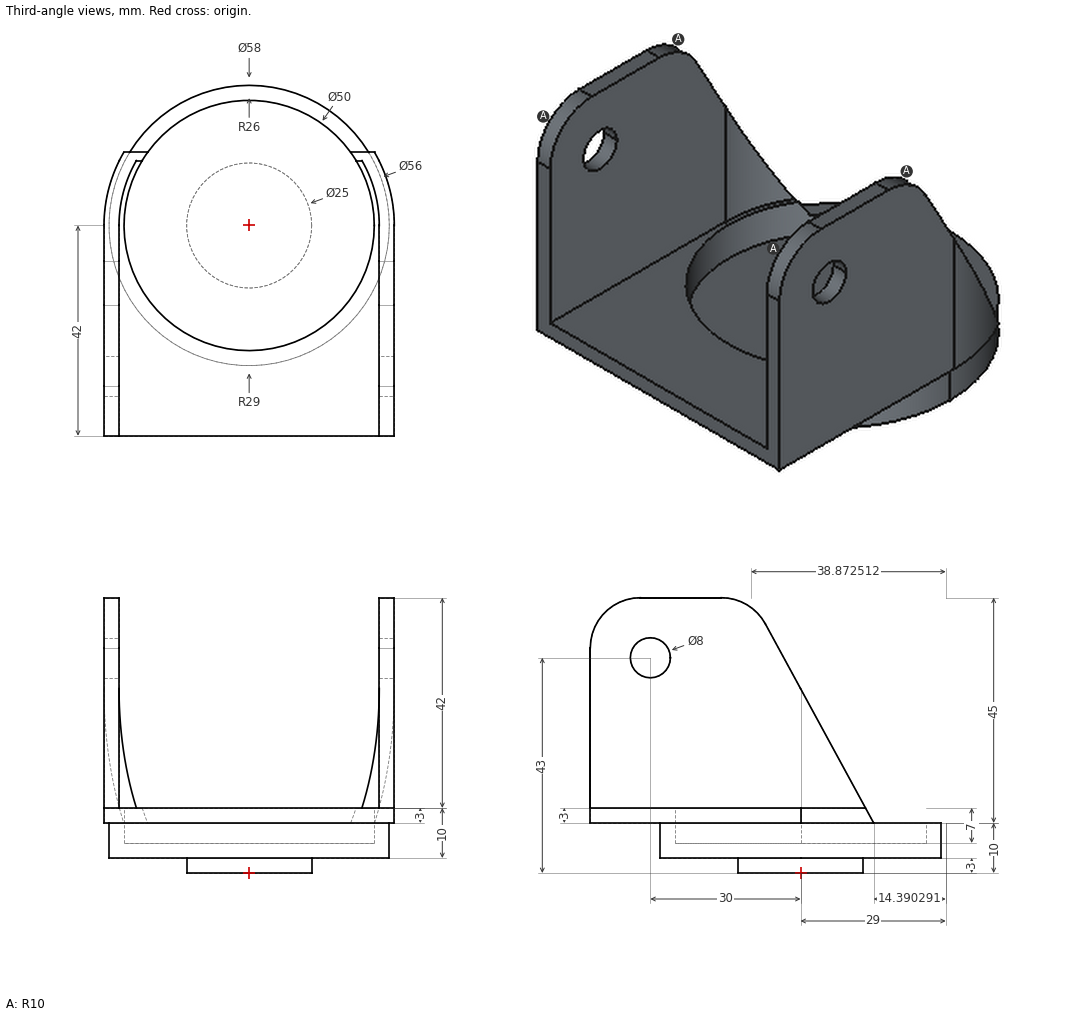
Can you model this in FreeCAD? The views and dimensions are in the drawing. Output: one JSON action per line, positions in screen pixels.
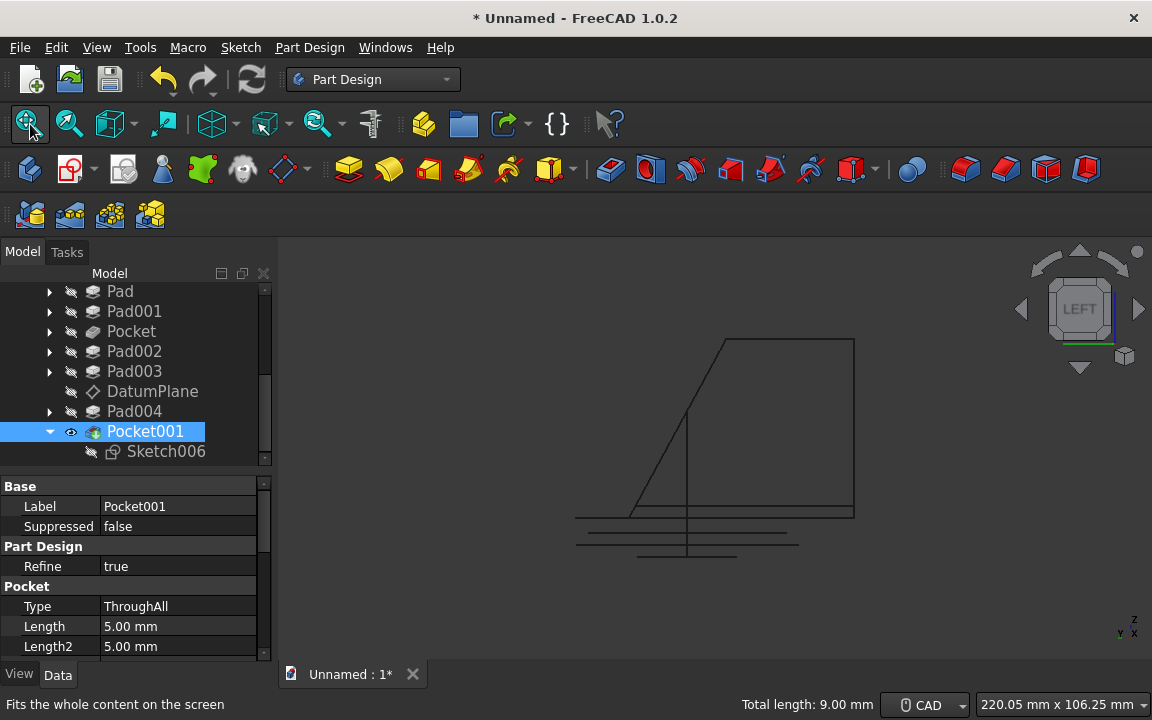
{"action": "key", "text": "0"}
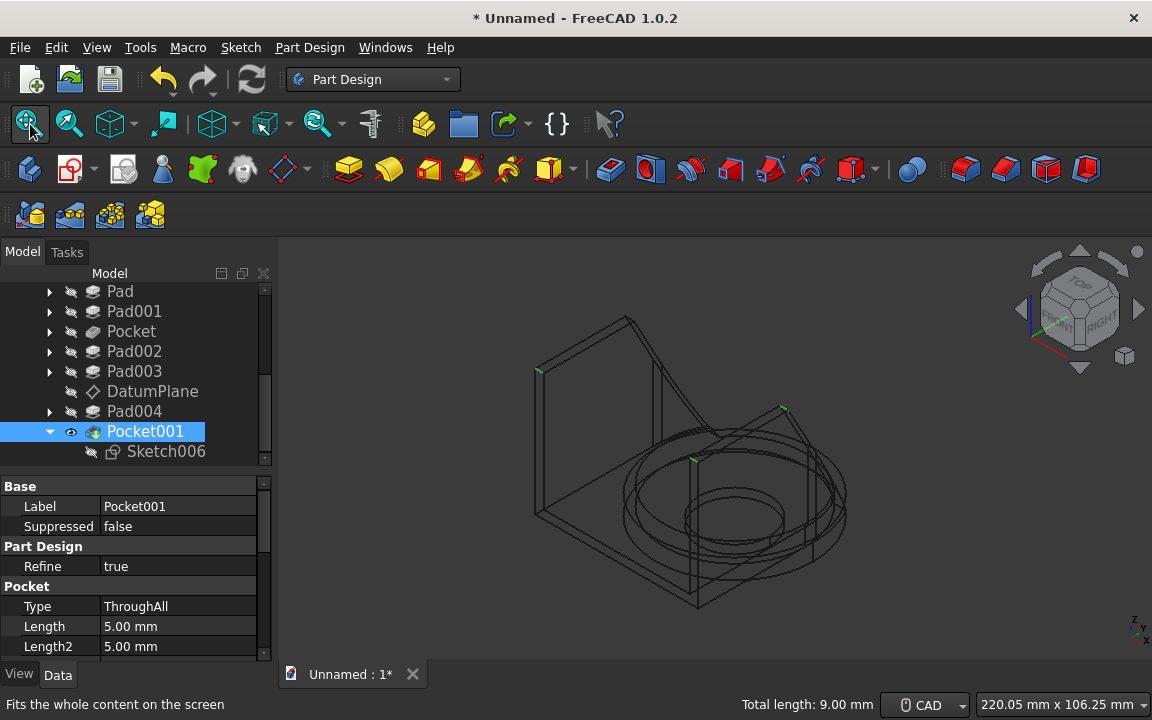
{"action": "left_click", "coordinate": [627, 316], "text": "ctrl"}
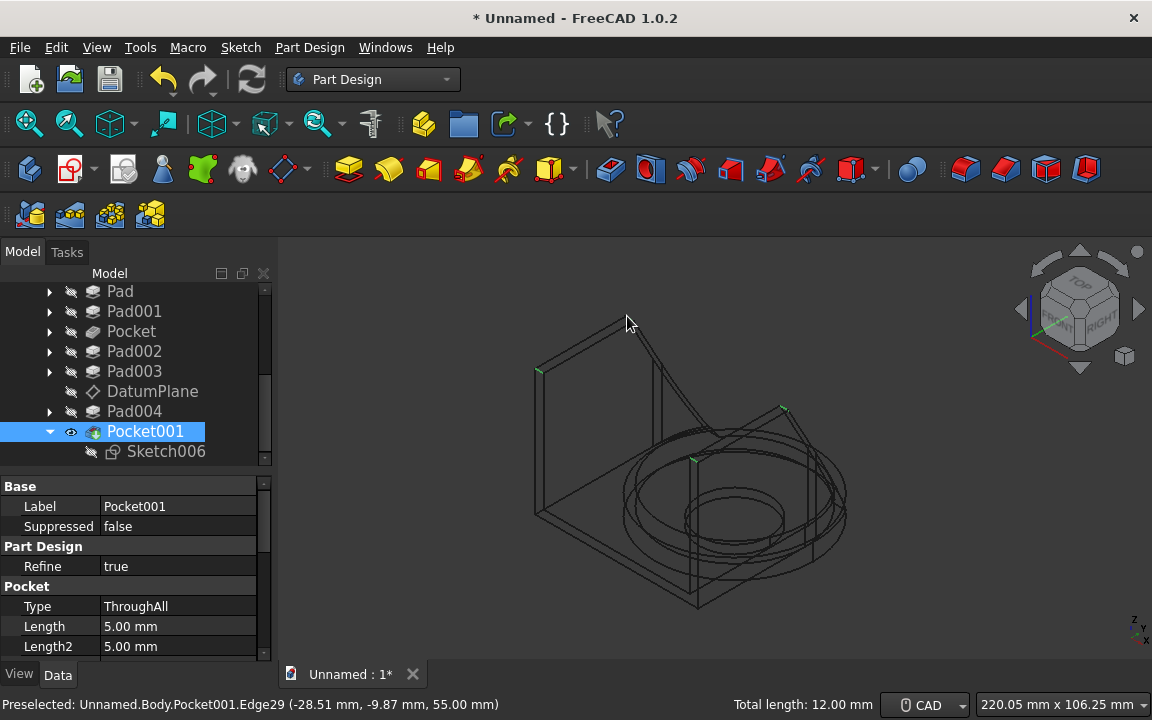
{"action": "key", "text": "v 1"}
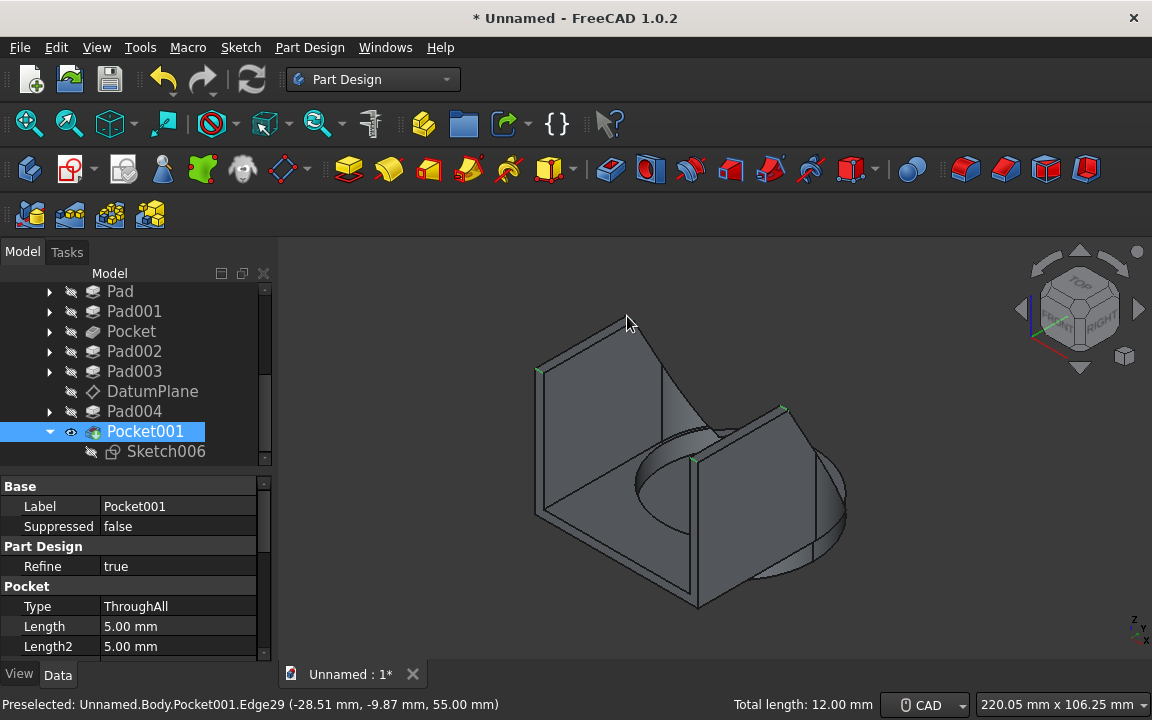
{"action": "left_click", "coordinate": [966, 170]}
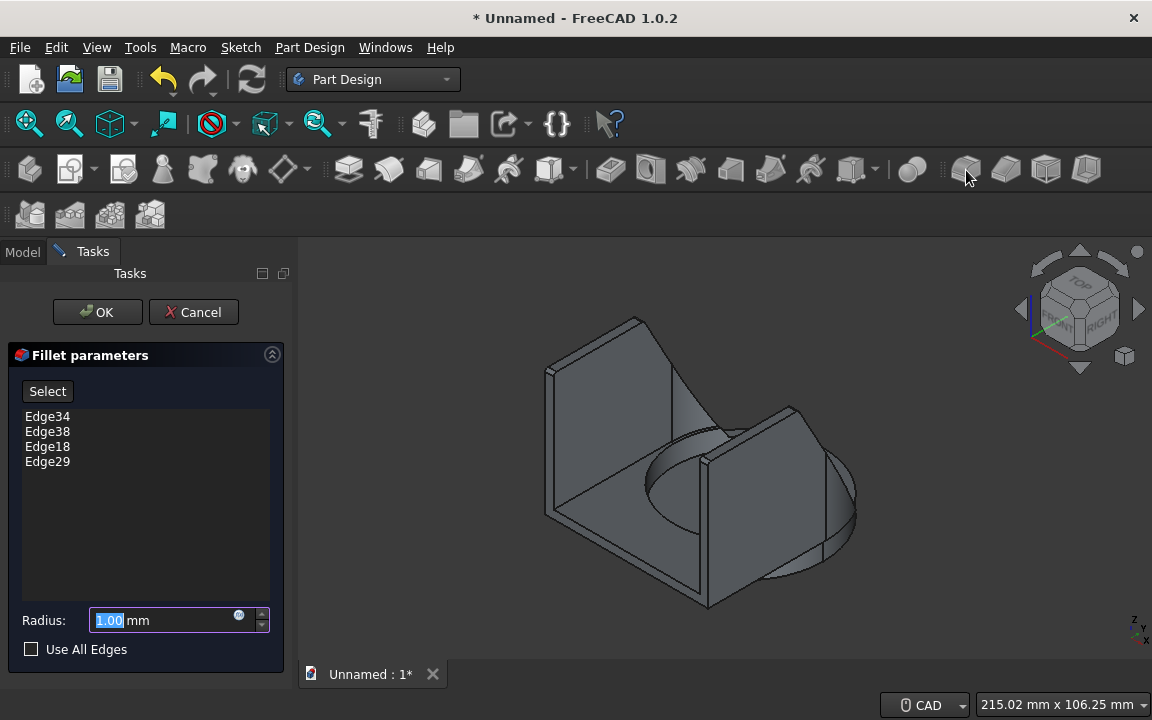
{"action": "type", "text": "10"}
{"action": "key", "text": "Tab"}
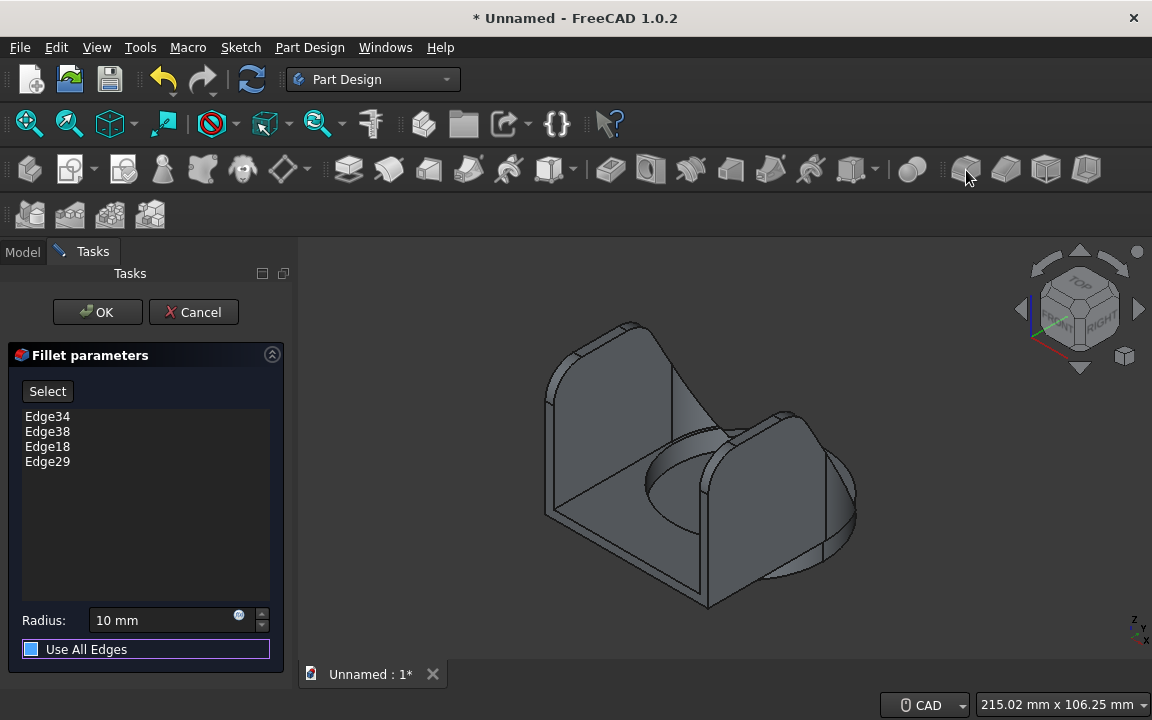
{"action": "left_click", "coordinate": [98, 312]}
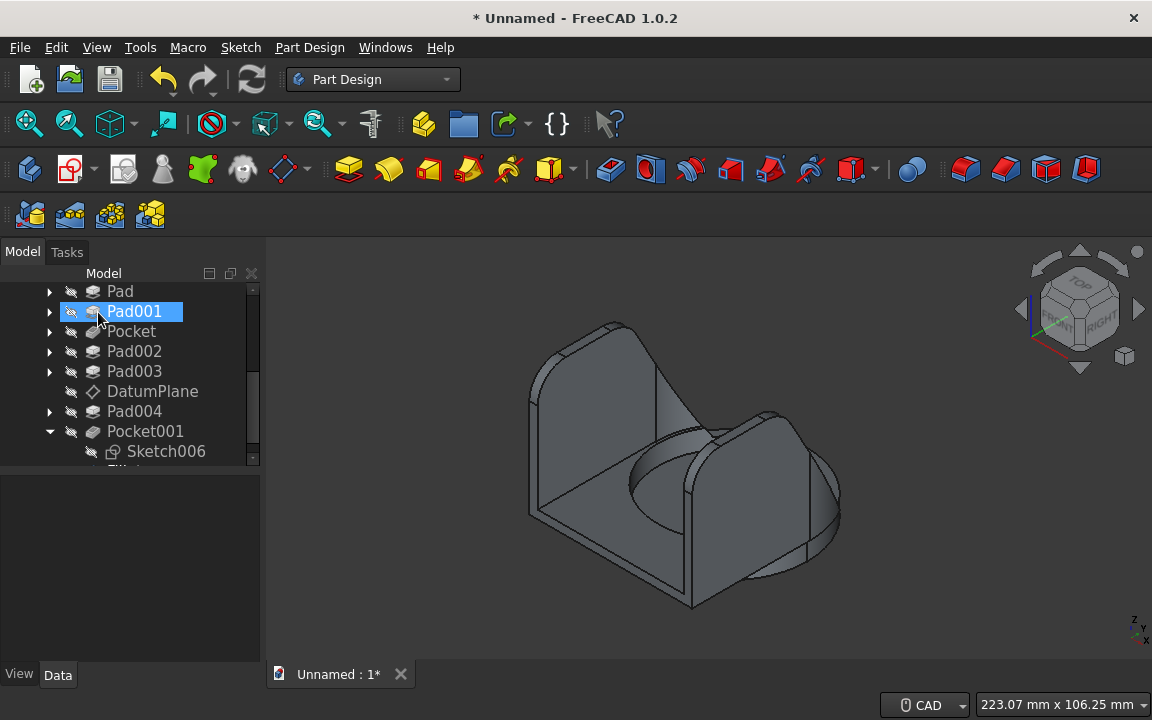
{"action": "left_click", "coordinate": [751, 501]}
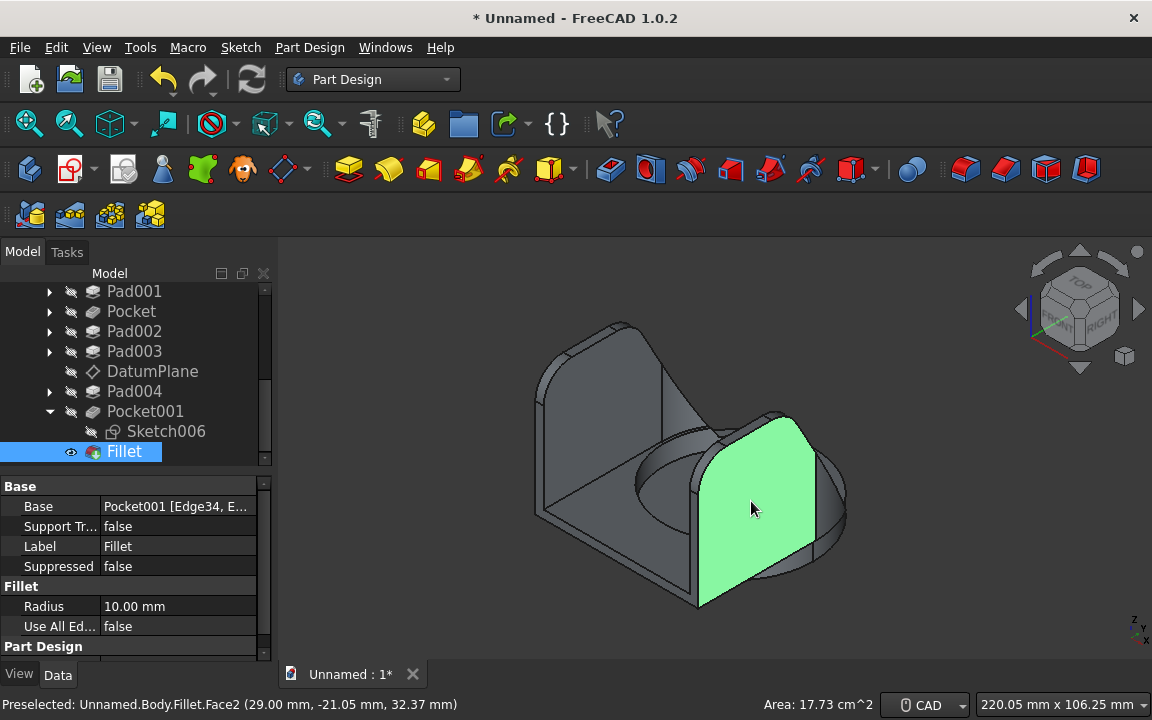
{"action": "left_click", "coordinate": [70, 170]}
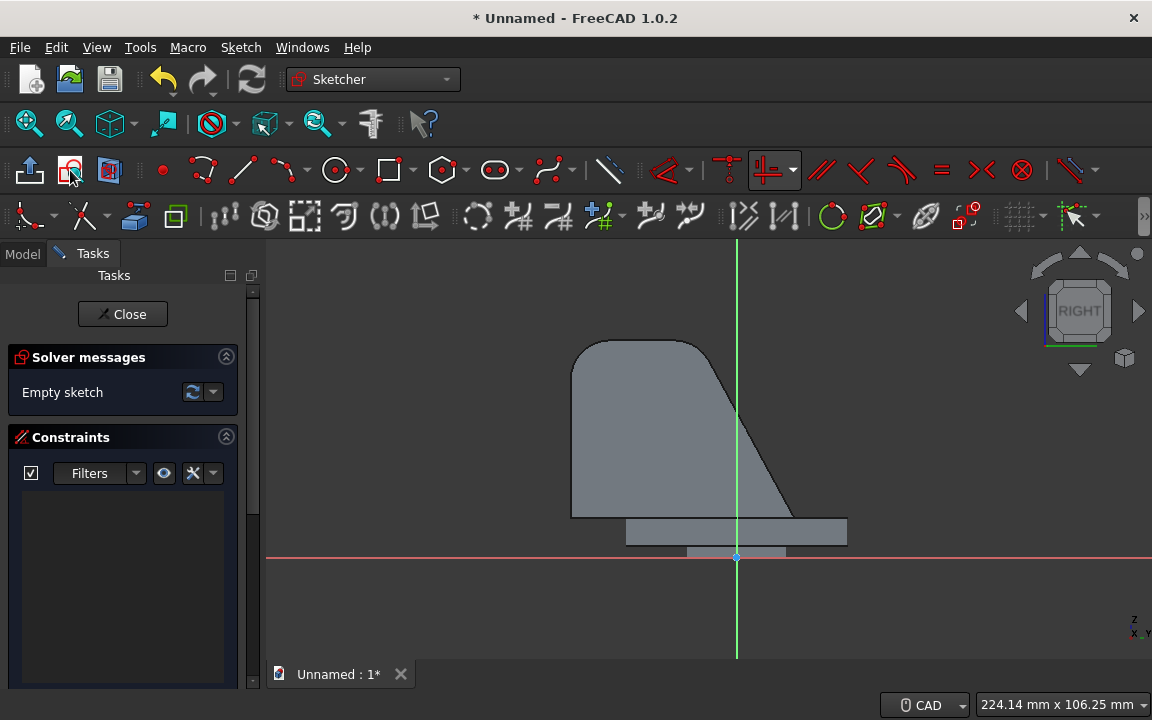
{"action": "scroll", "coordinate": [615, 378], "scroll_direction": "up", "scroll_amount": 10}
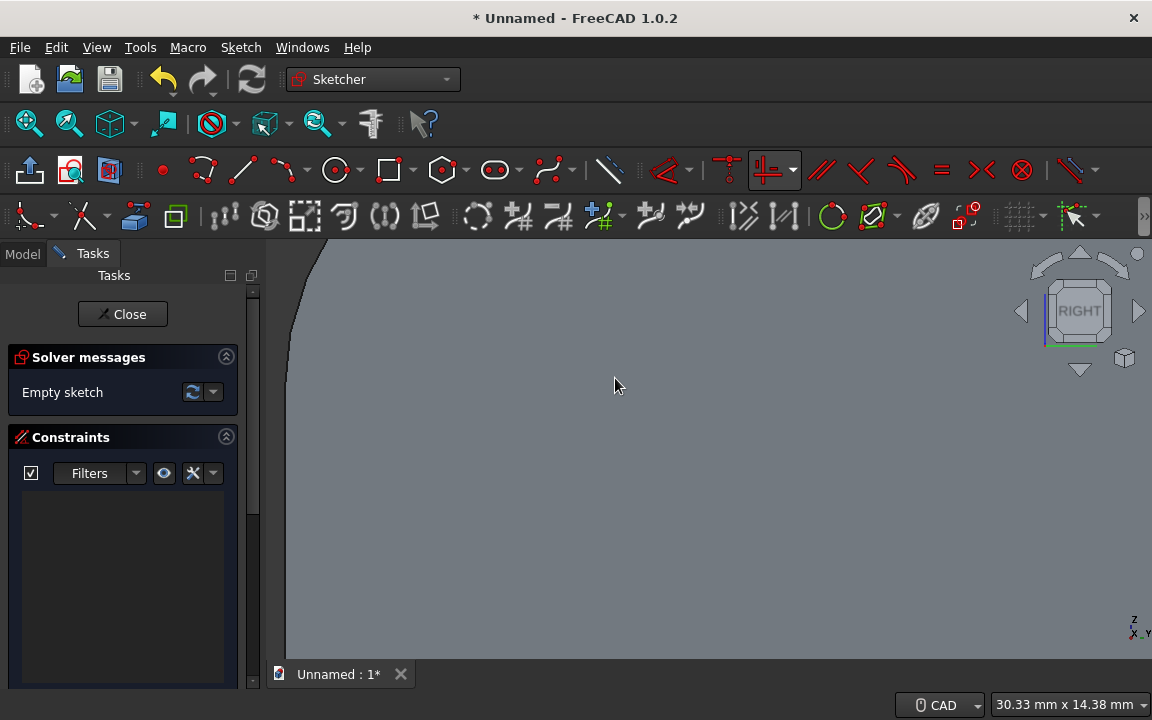
{"action": "left_click", "coordinate": [336, 170]}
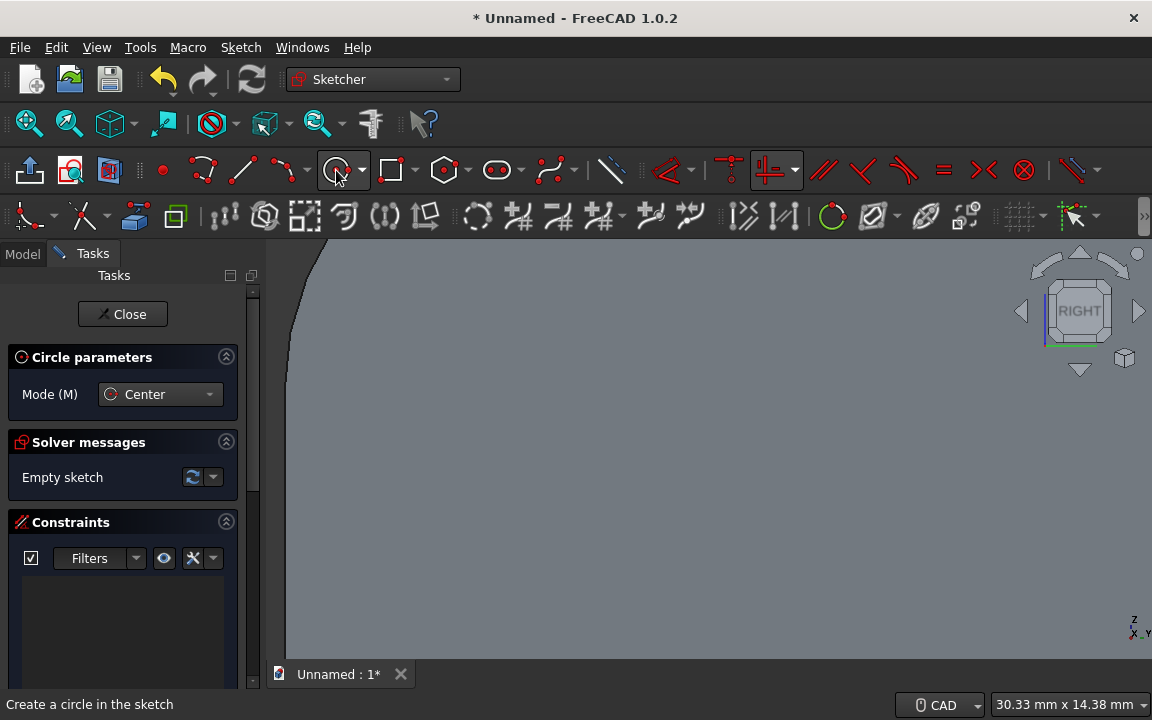
{"action": "left_click", "coordinate": [635, 448]}
{"action": "left_click", "coordinate": [718, 365]}
{"action": "key", "text": "Escape"}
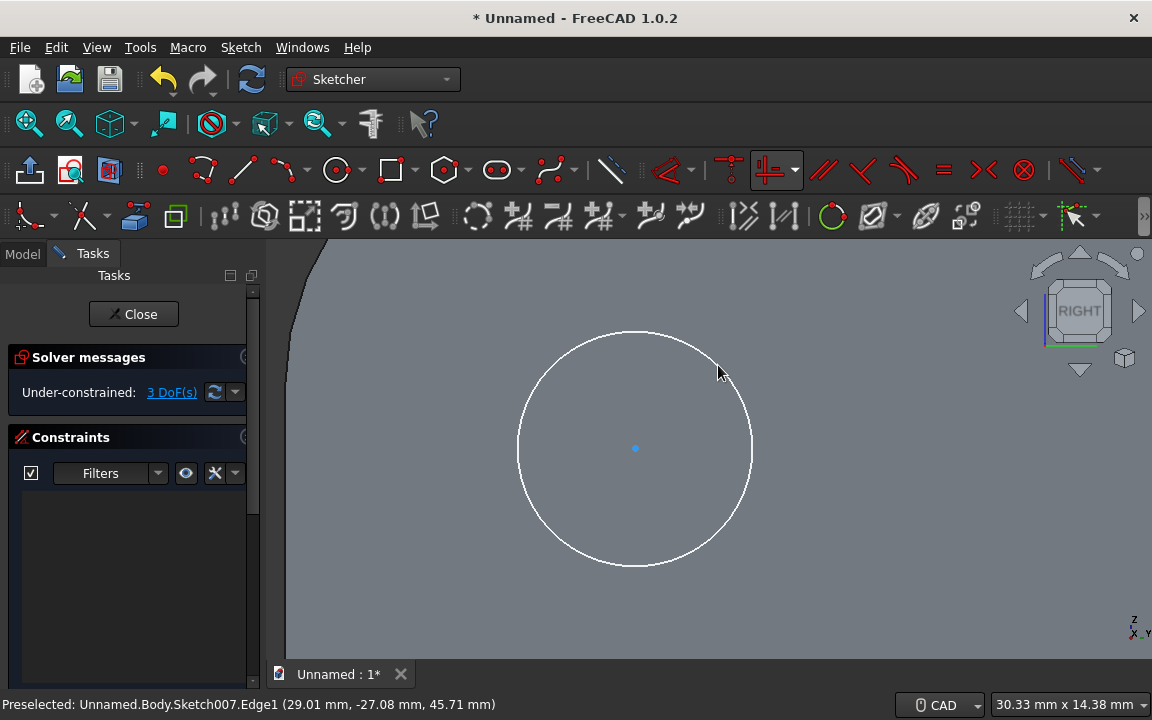
{"action": "left_click", "coordinate": [666, 170]}